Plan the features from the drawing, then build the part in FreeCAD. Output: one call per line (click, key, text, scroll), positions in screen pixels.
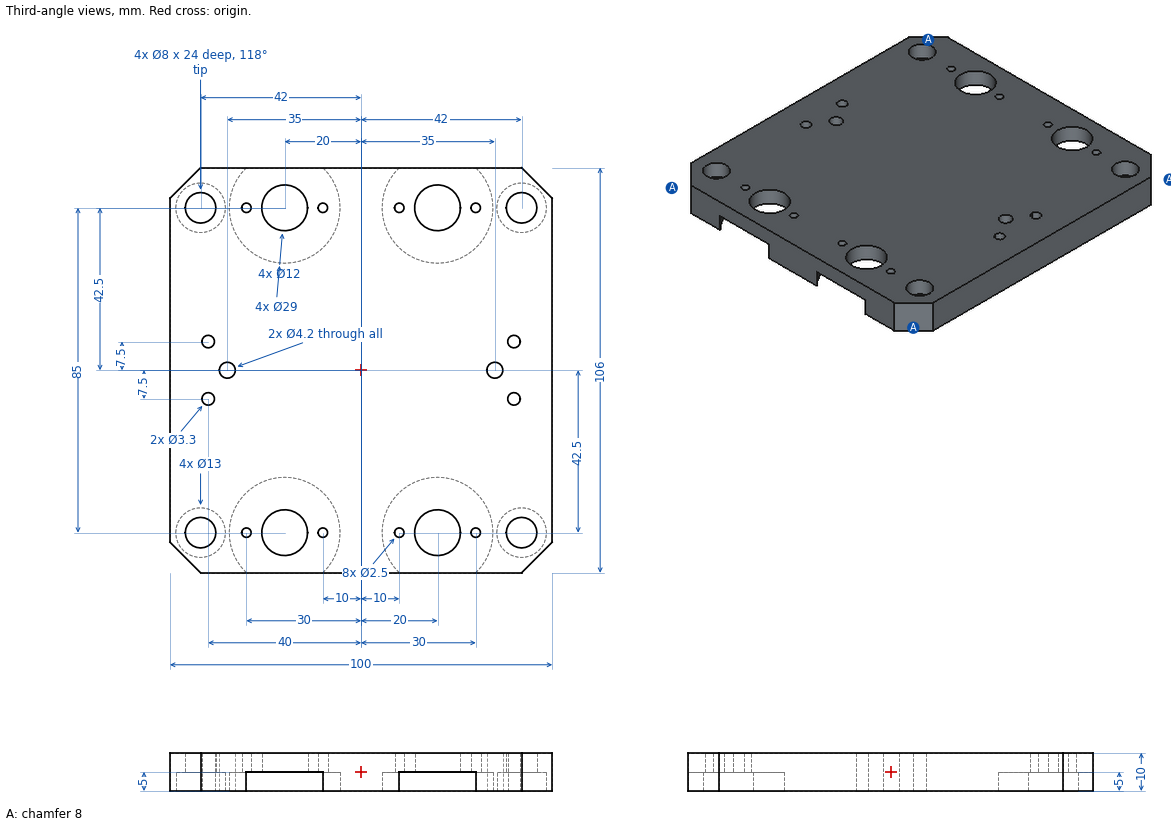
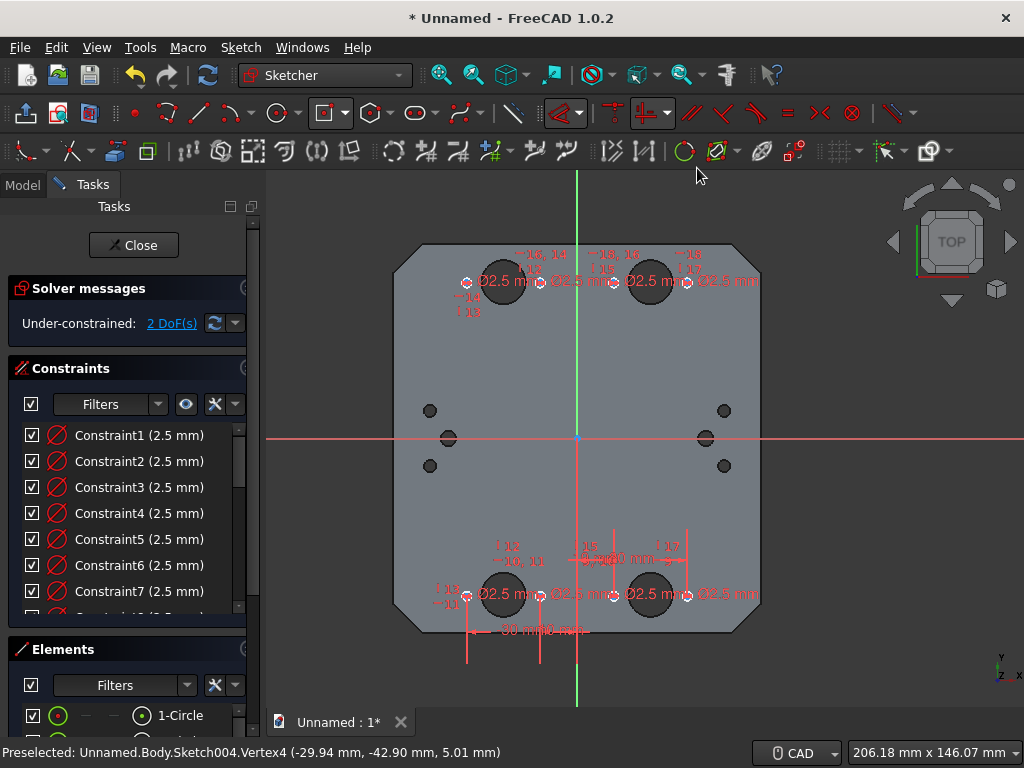
click(540, 596)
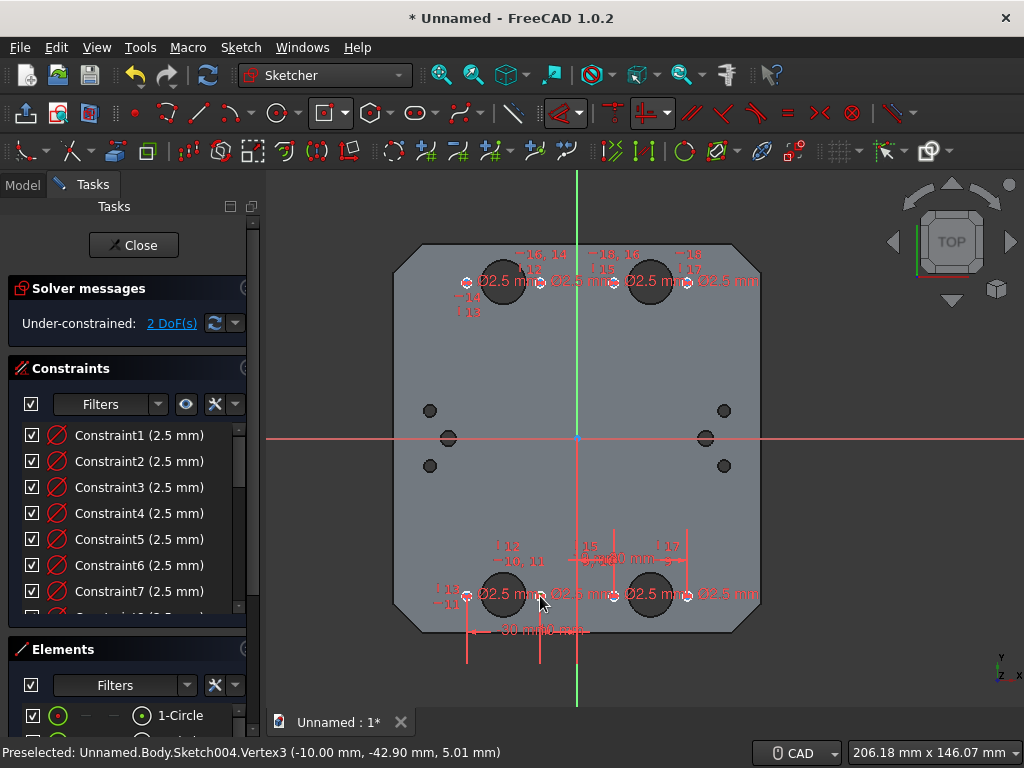
click(540, 283)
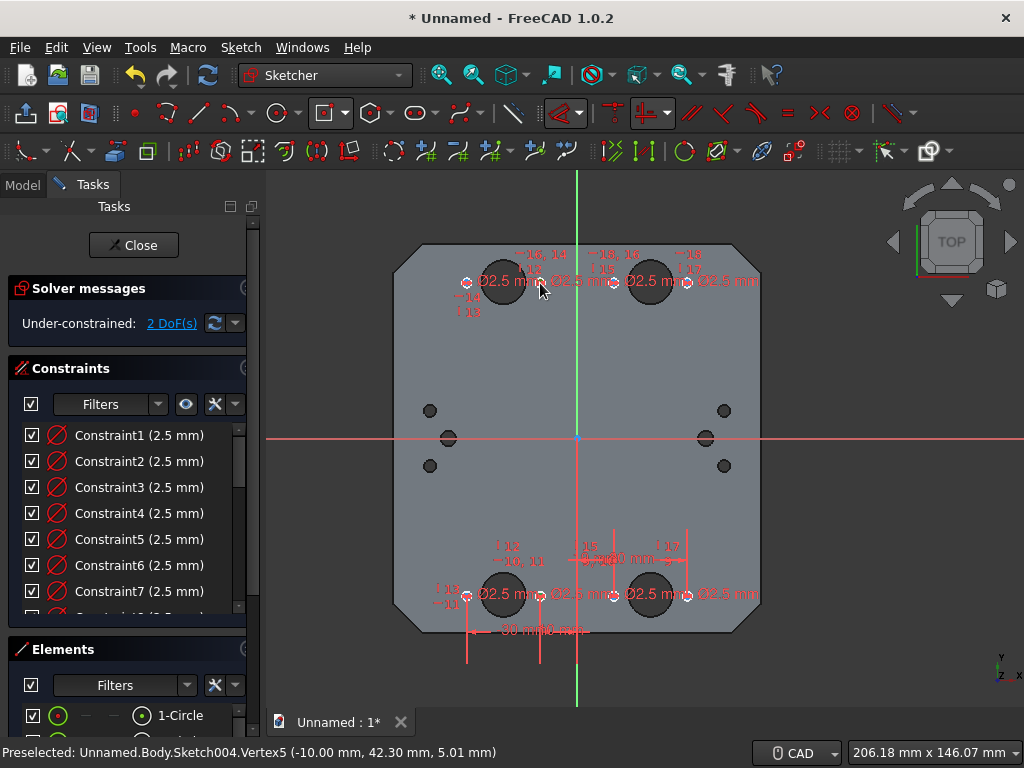
click(582, 114)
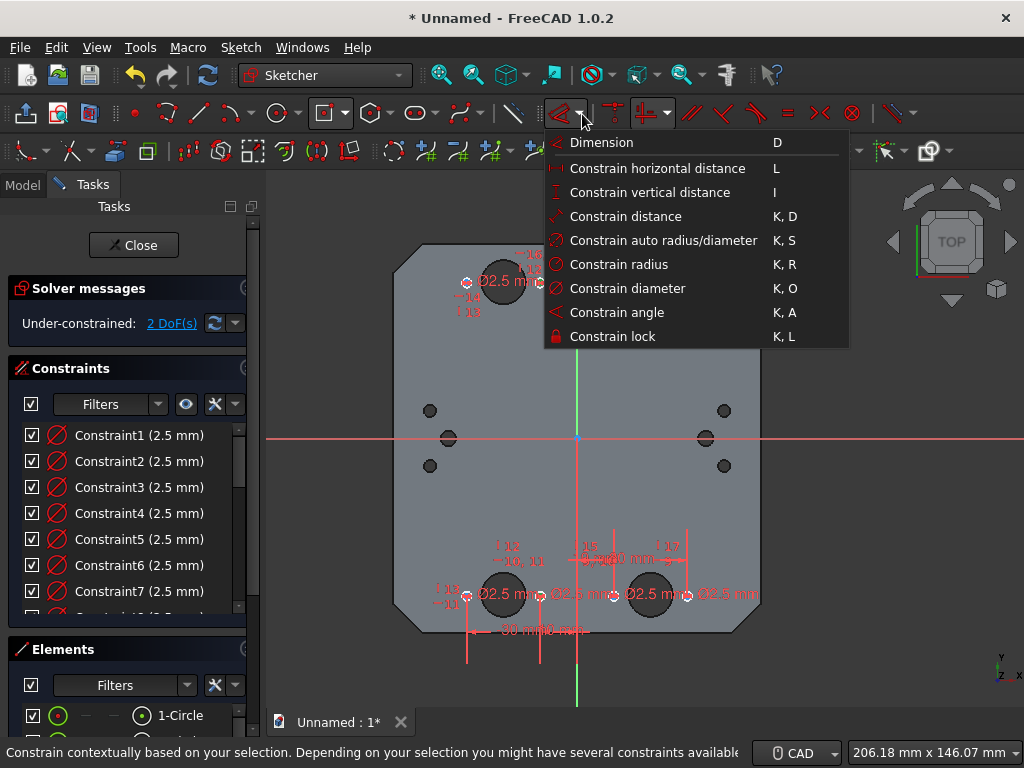
click(697, 192)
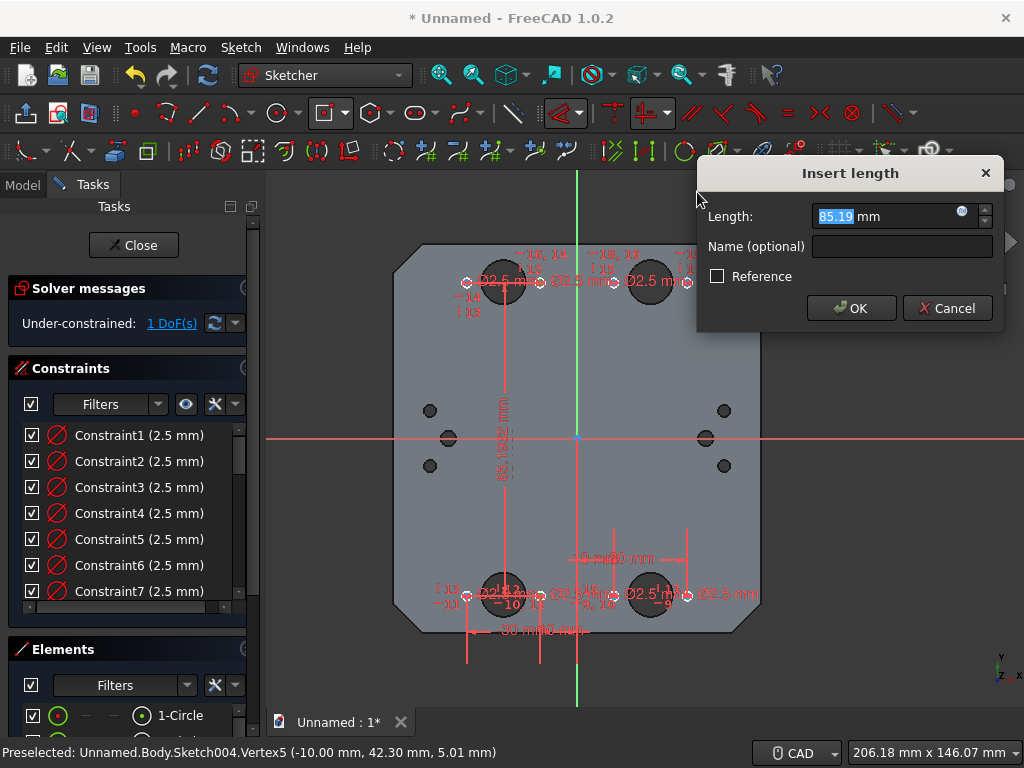
text(85)
key(Return)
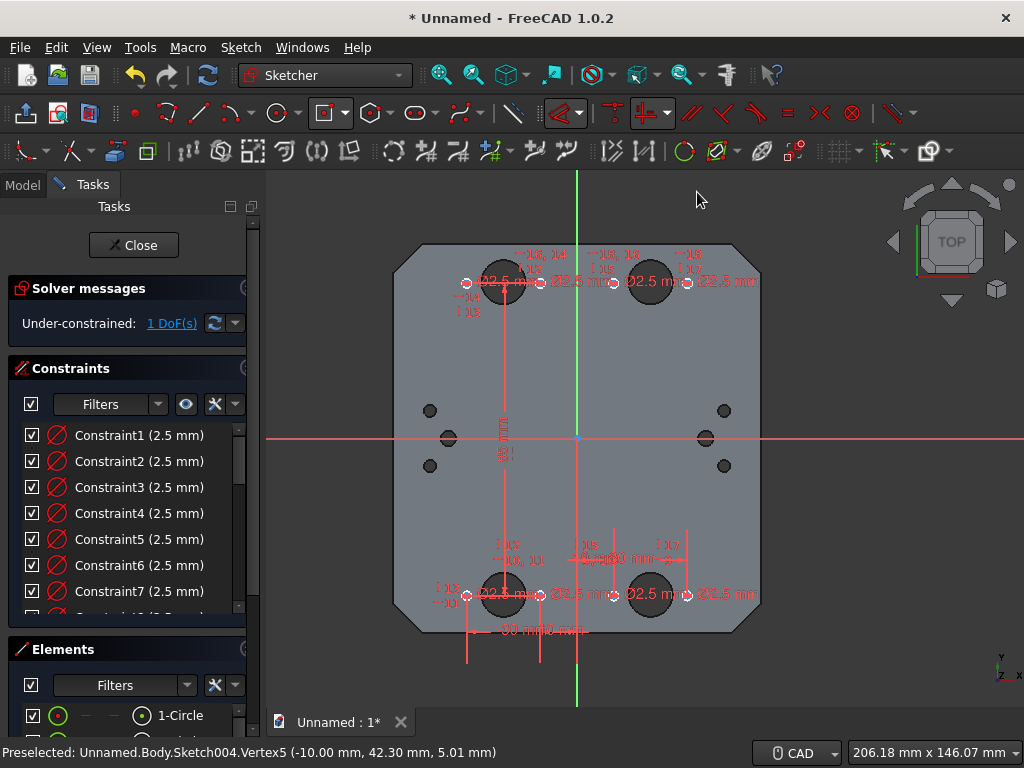
click(614, 596)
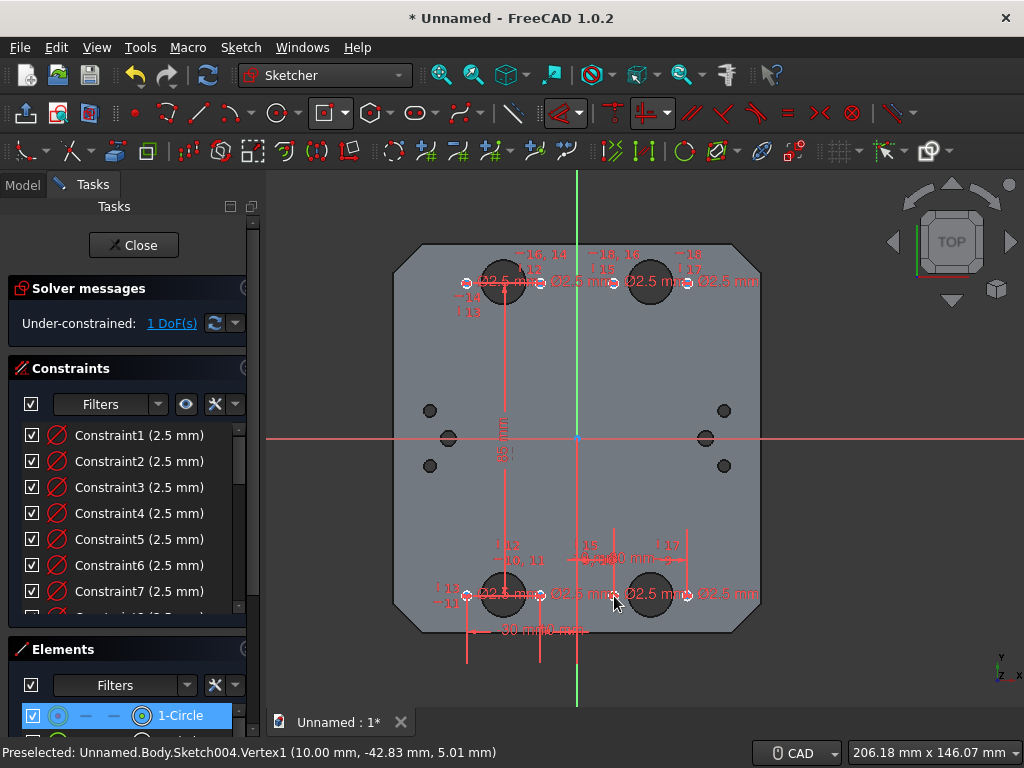
click(582, 114)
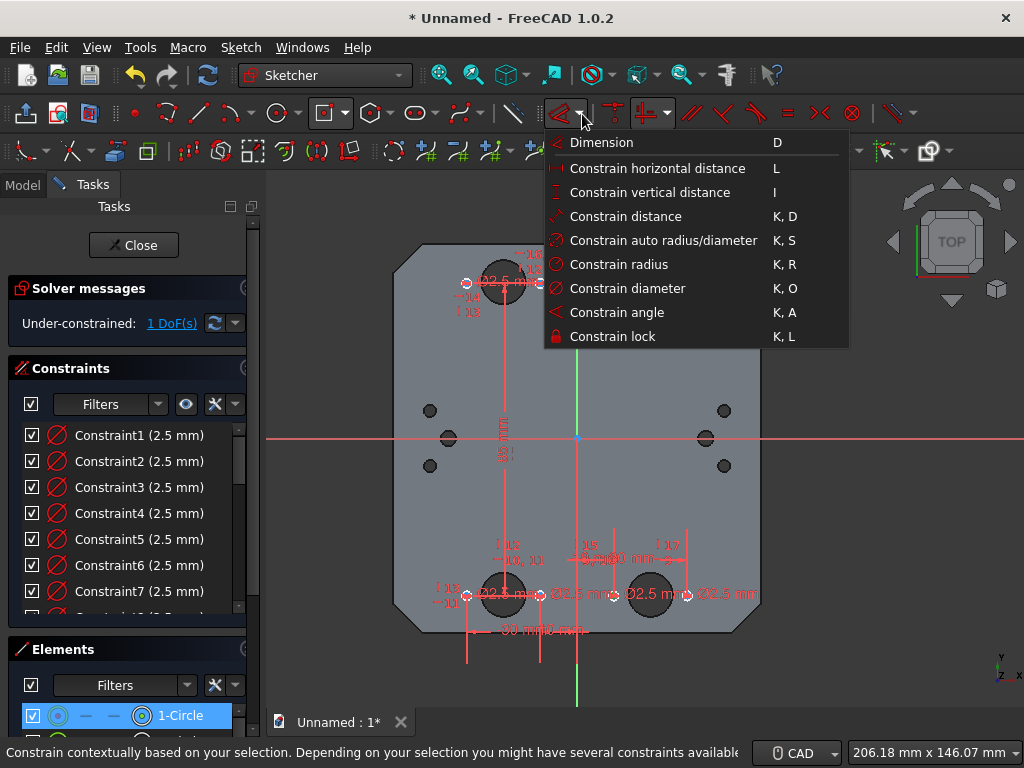
click(697, 192)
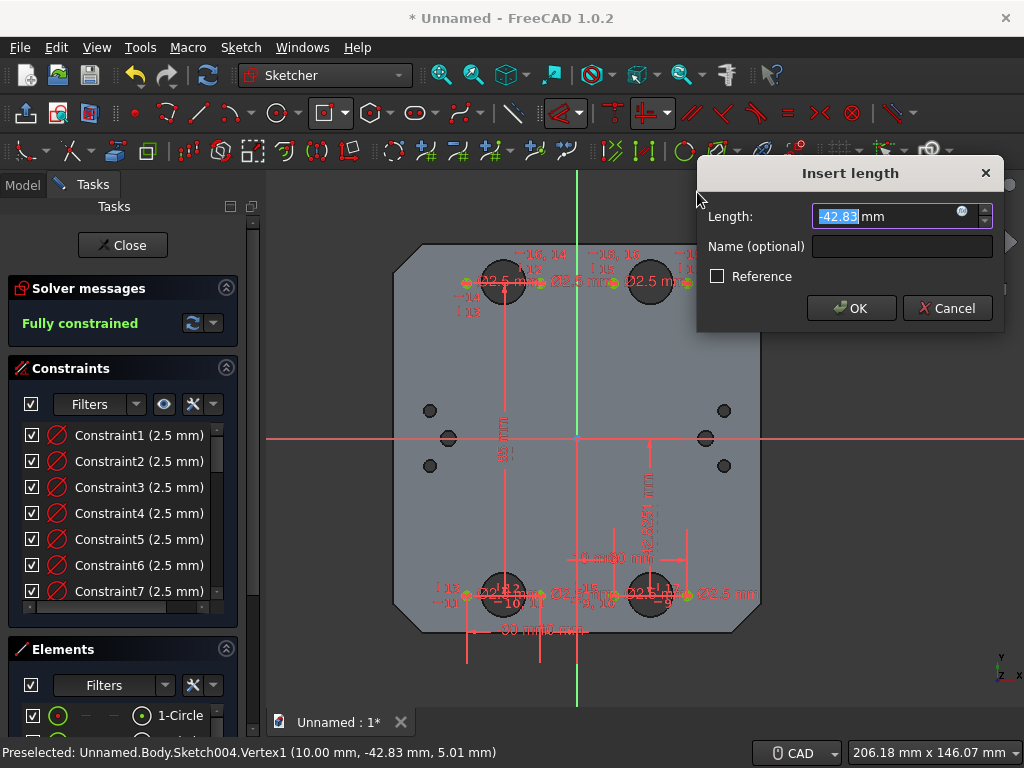
text(-42.5)
key(Return)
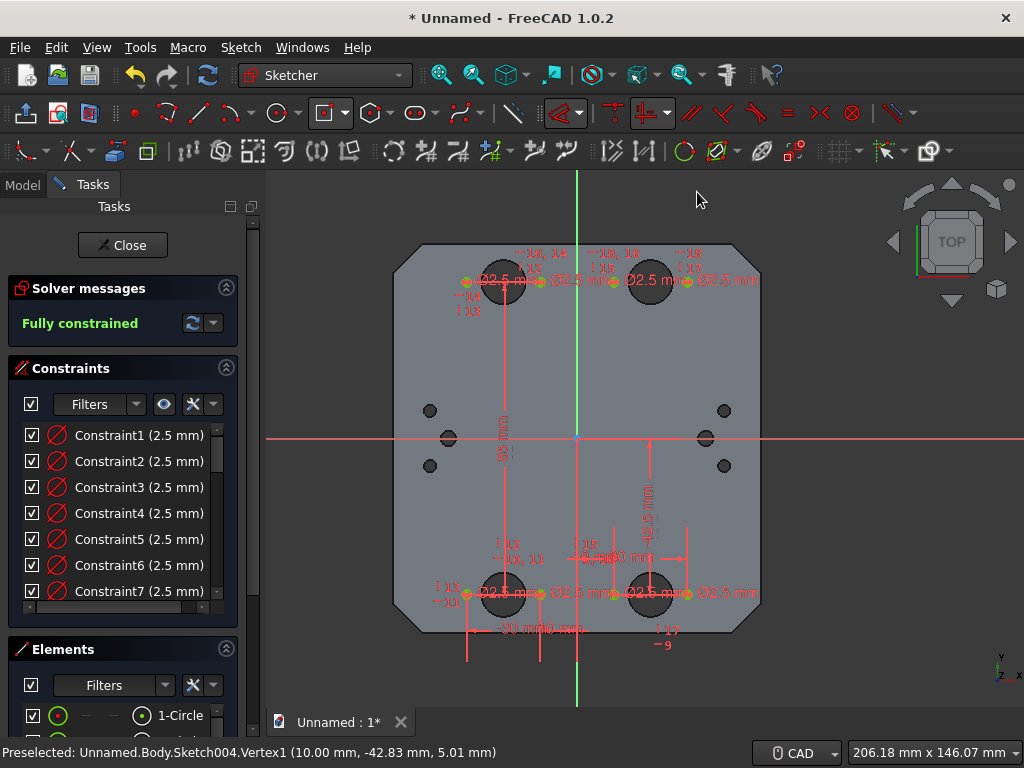
click(123, 245)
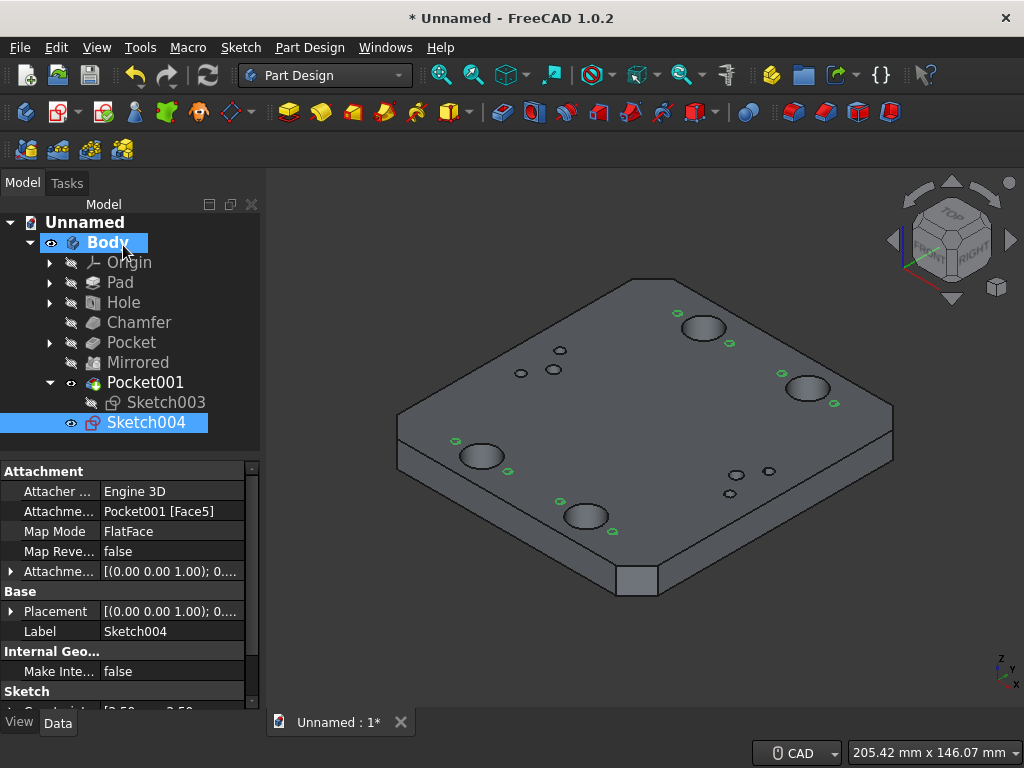
click(504, 112)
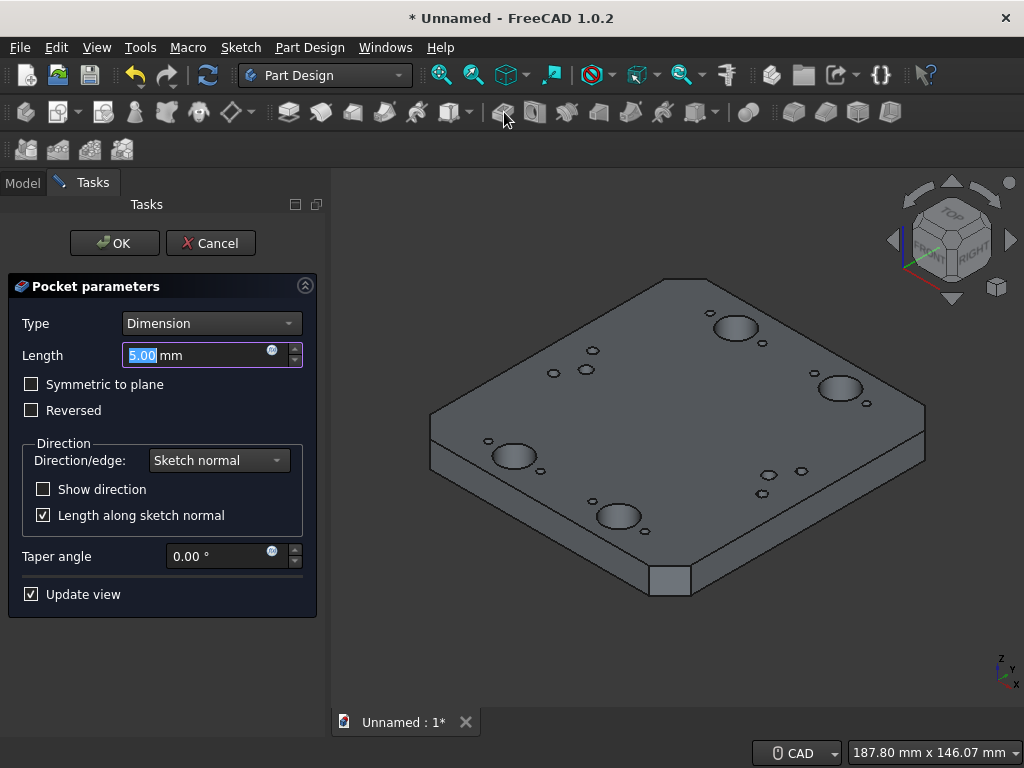
click(212, 324)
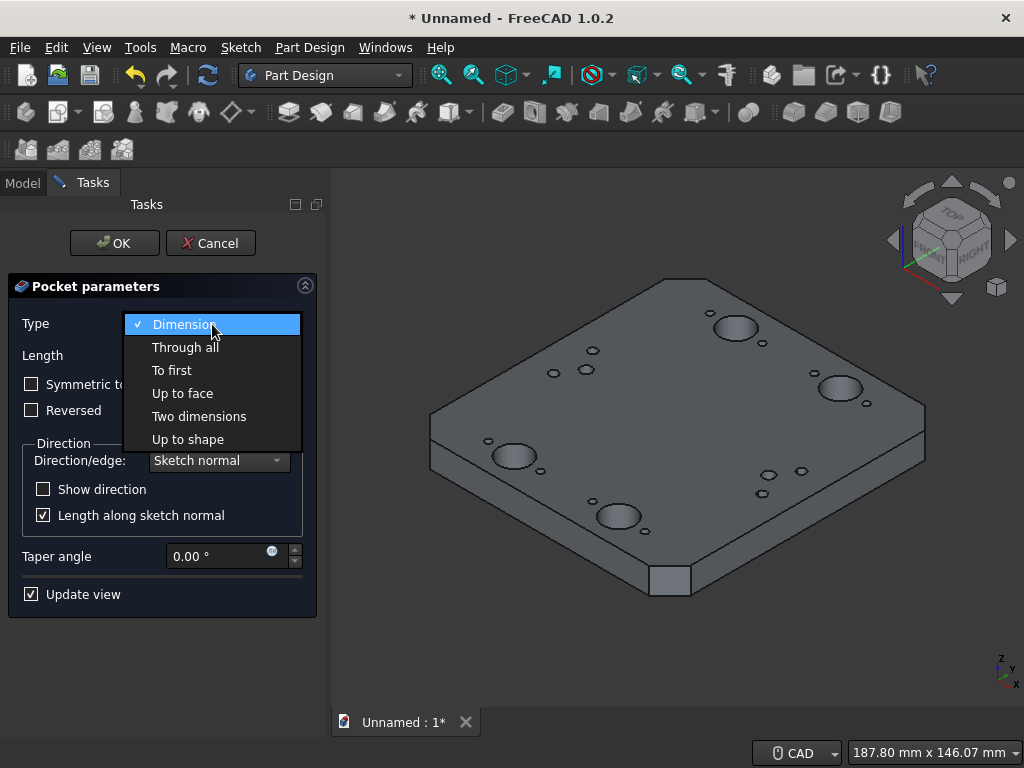
click(212, 348)